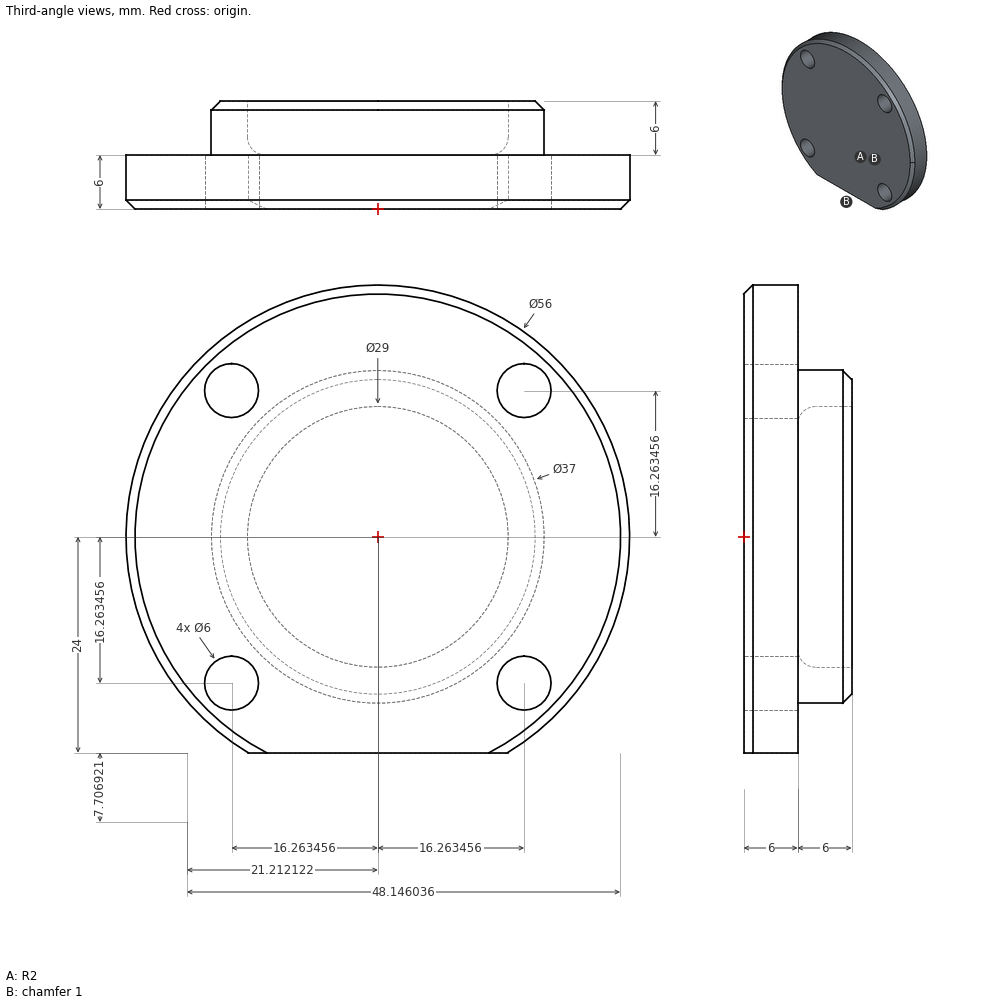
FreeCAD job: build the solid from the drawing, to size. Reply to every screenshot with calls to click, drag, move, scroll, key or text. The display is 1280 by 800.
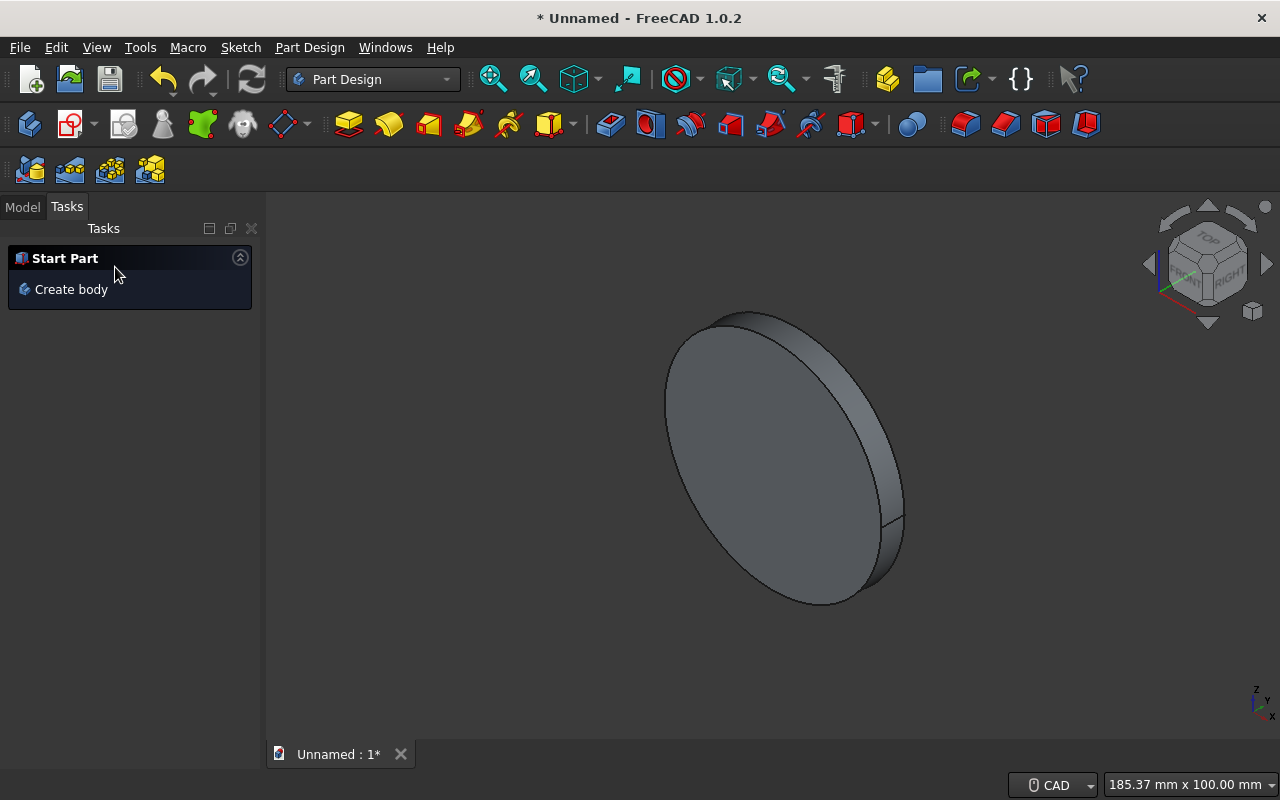
key(2)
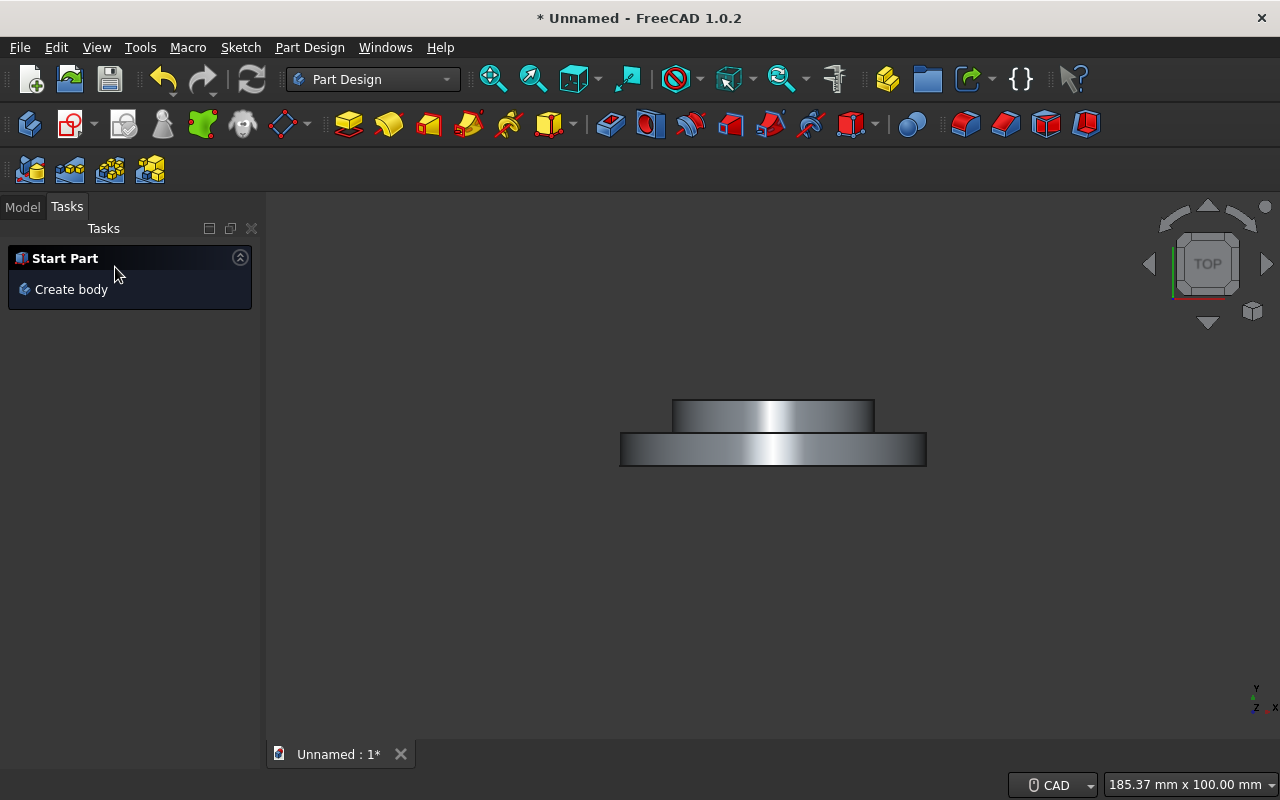
click(494, 80)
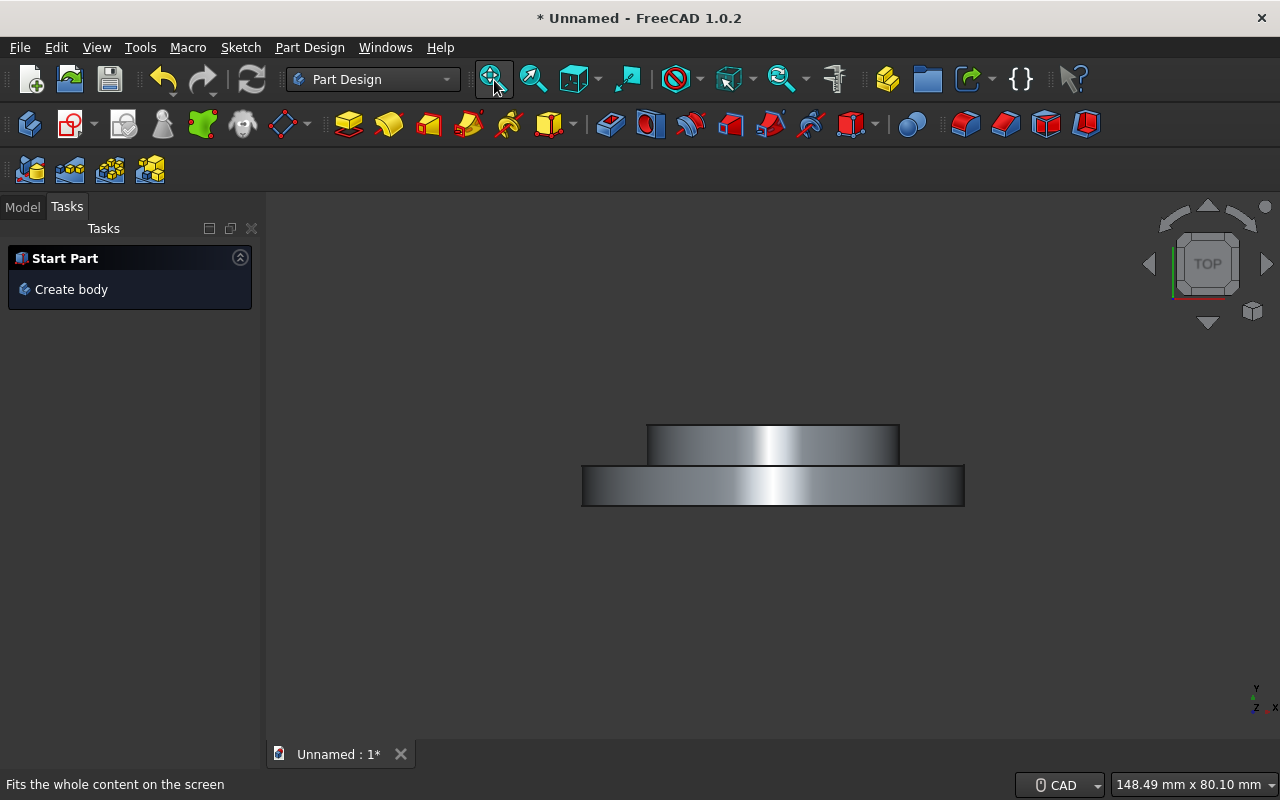
key(1)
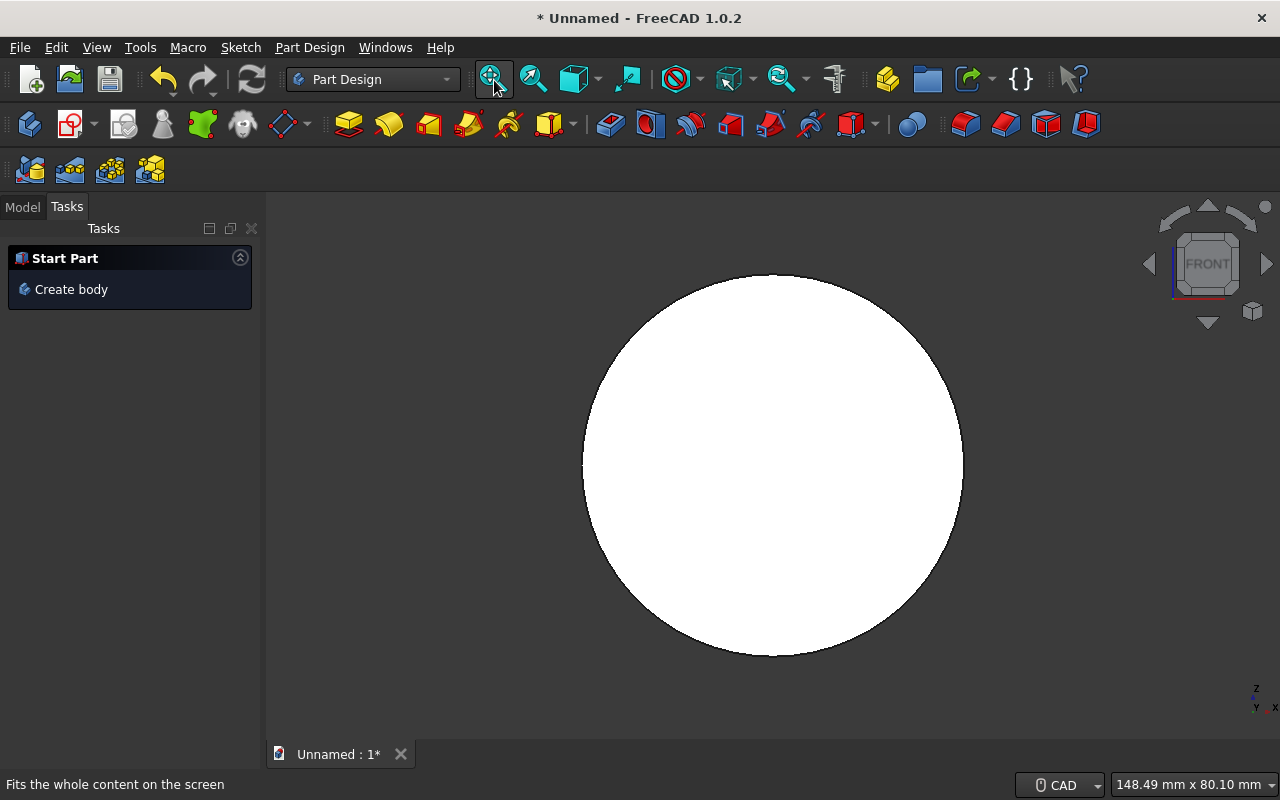
key(3)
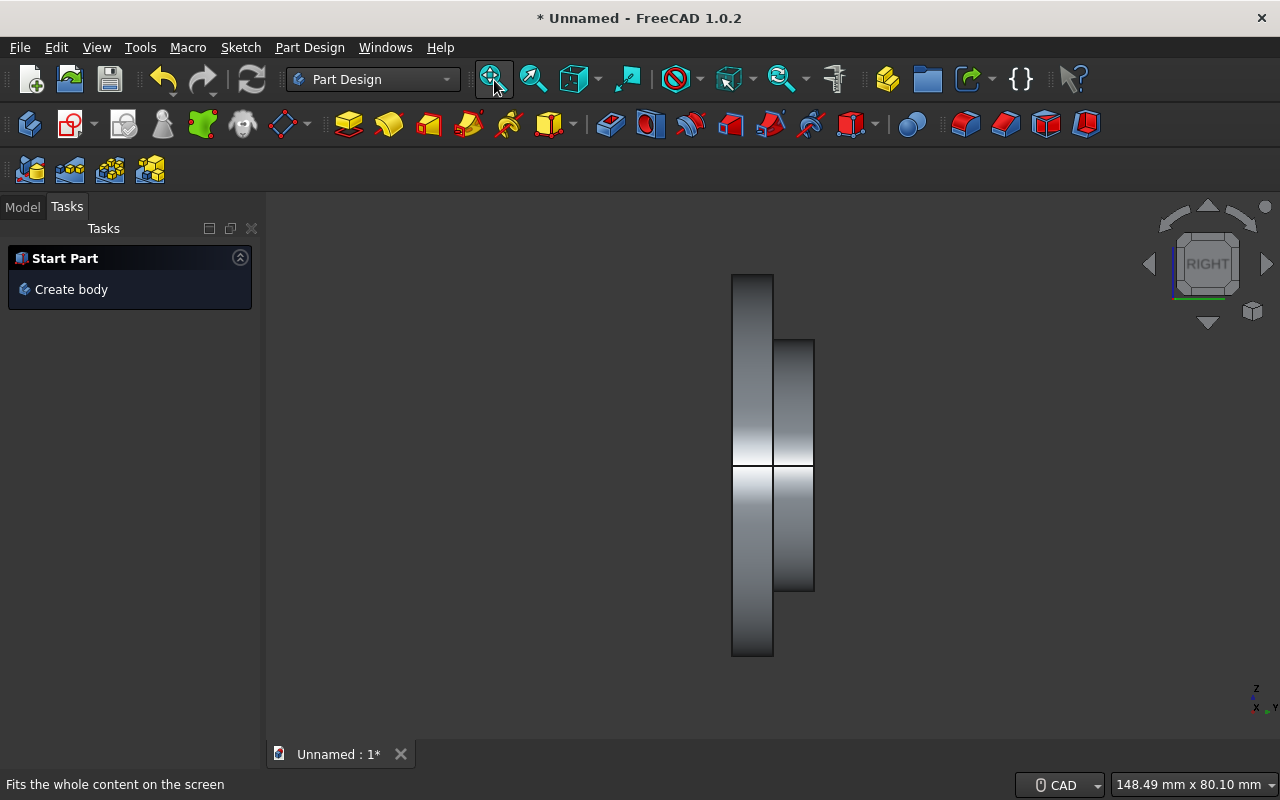
key(5)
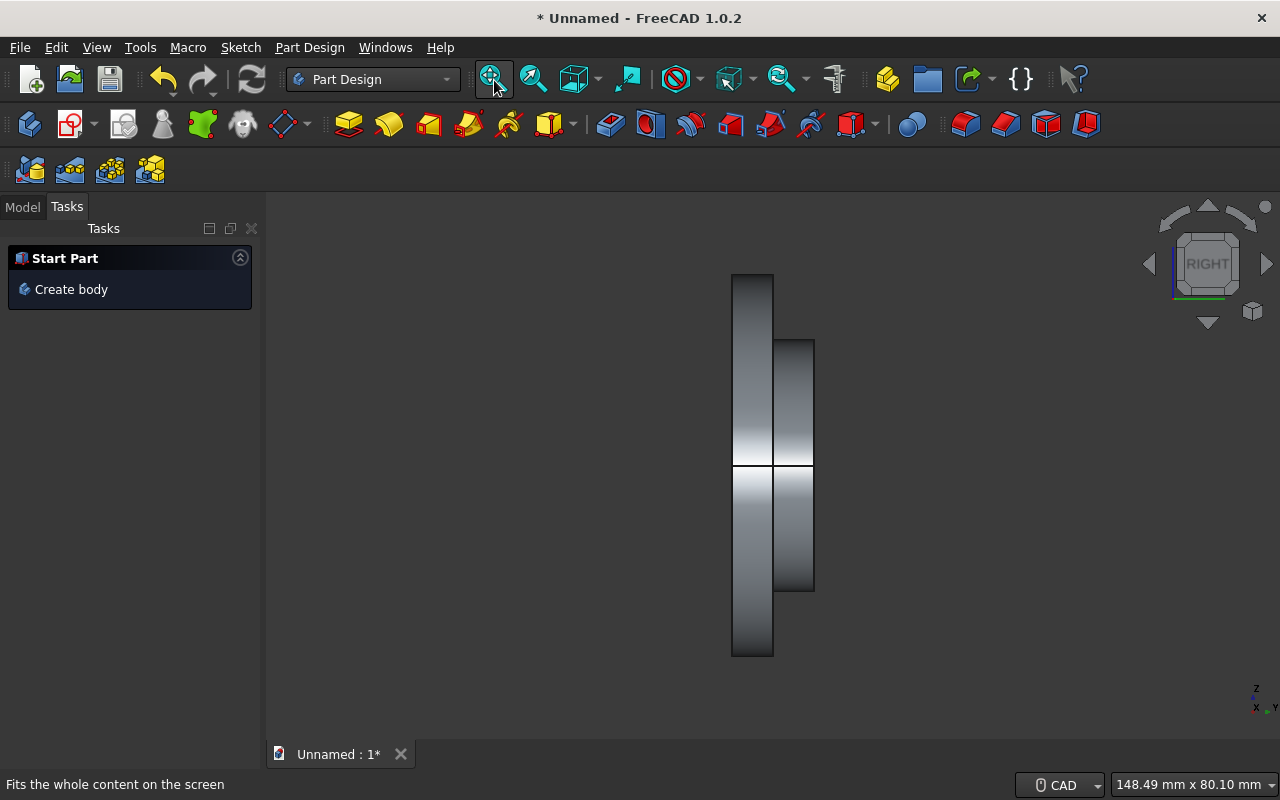
click(494, 80)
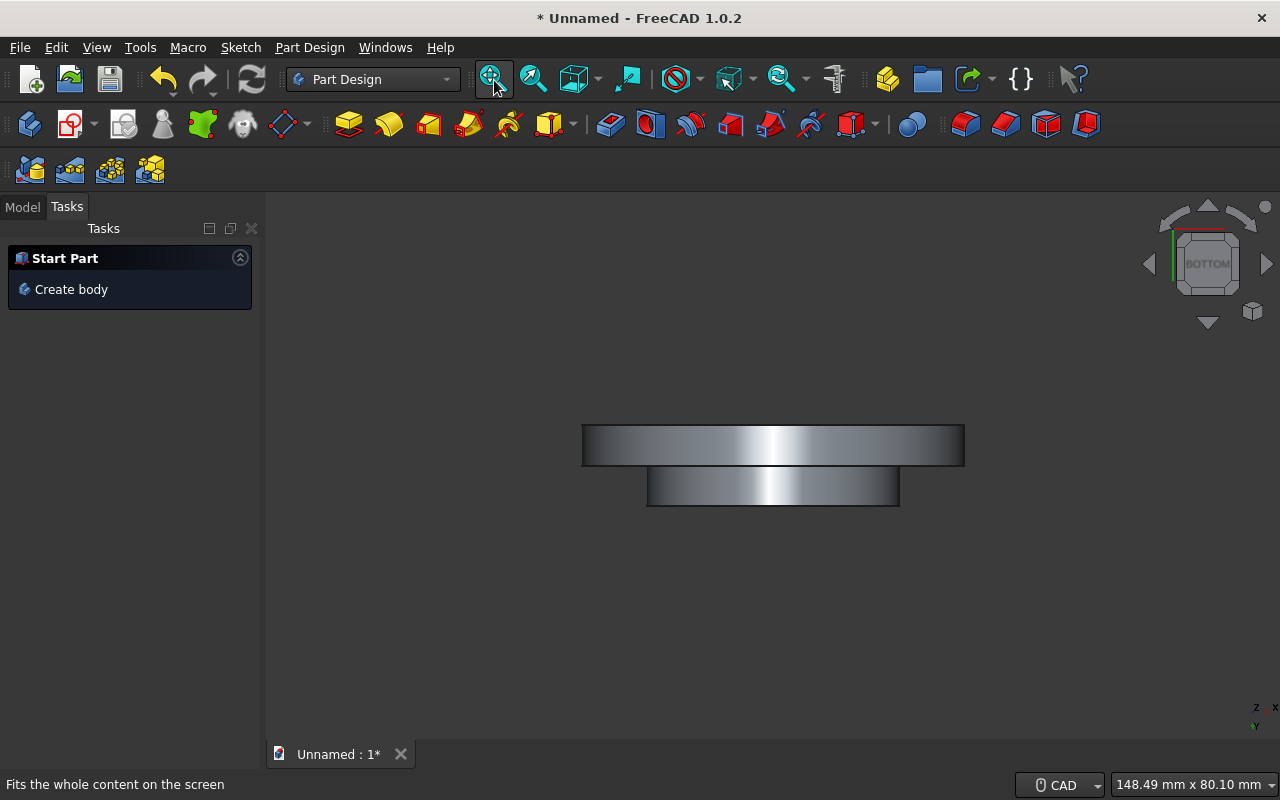
key(4)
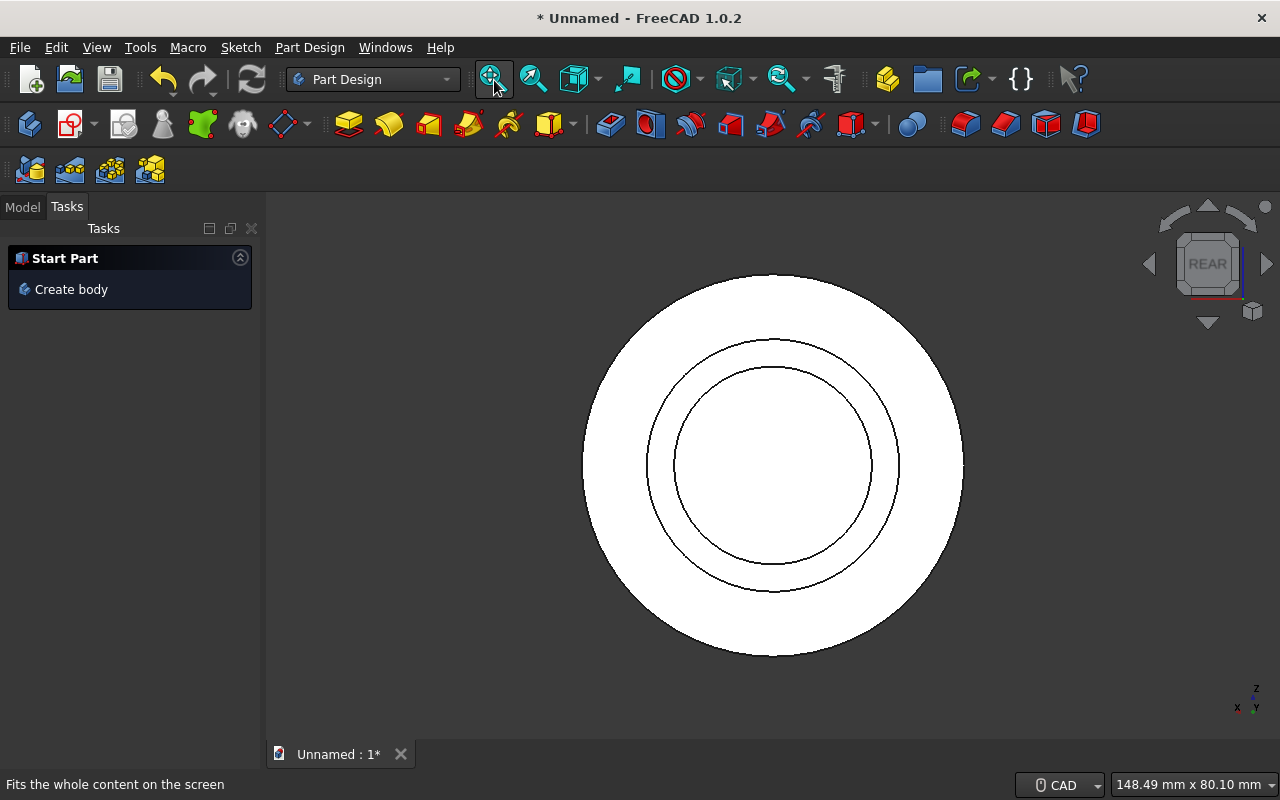
key(6)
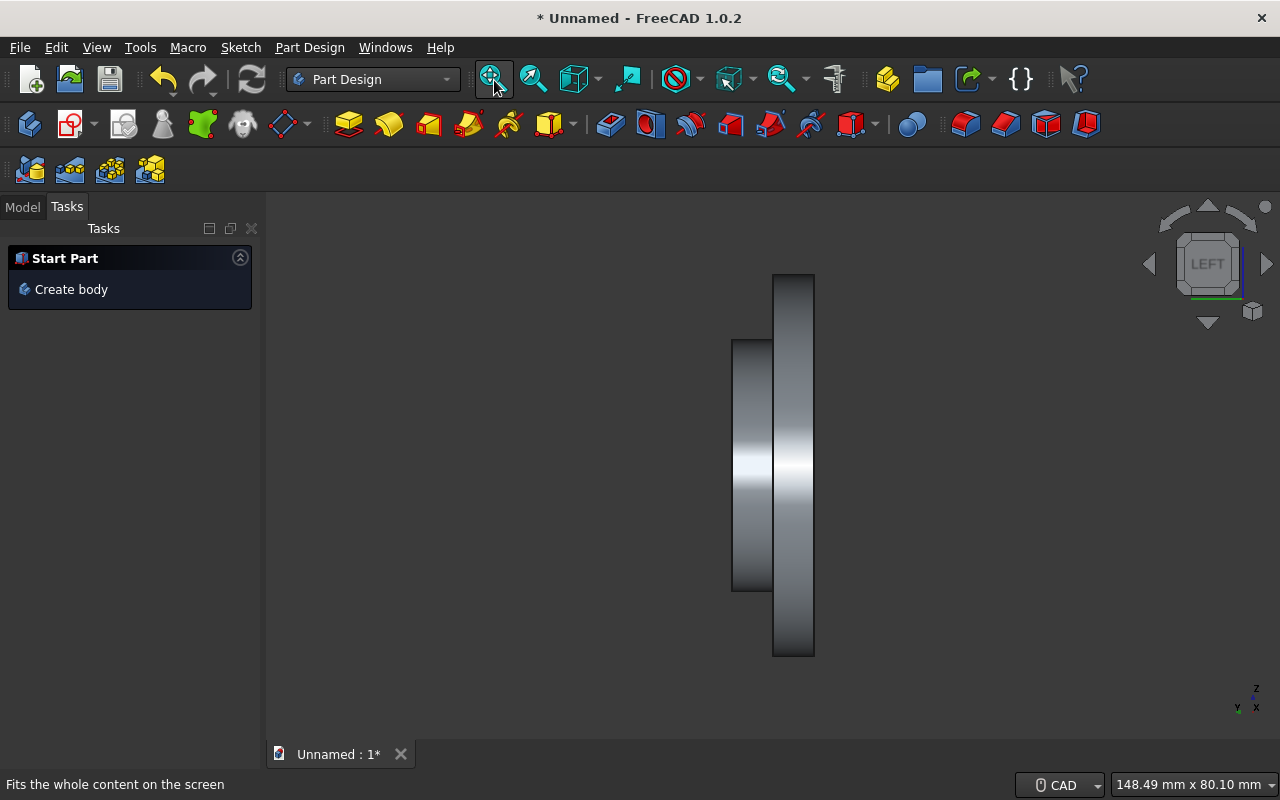
key(v)
key(3)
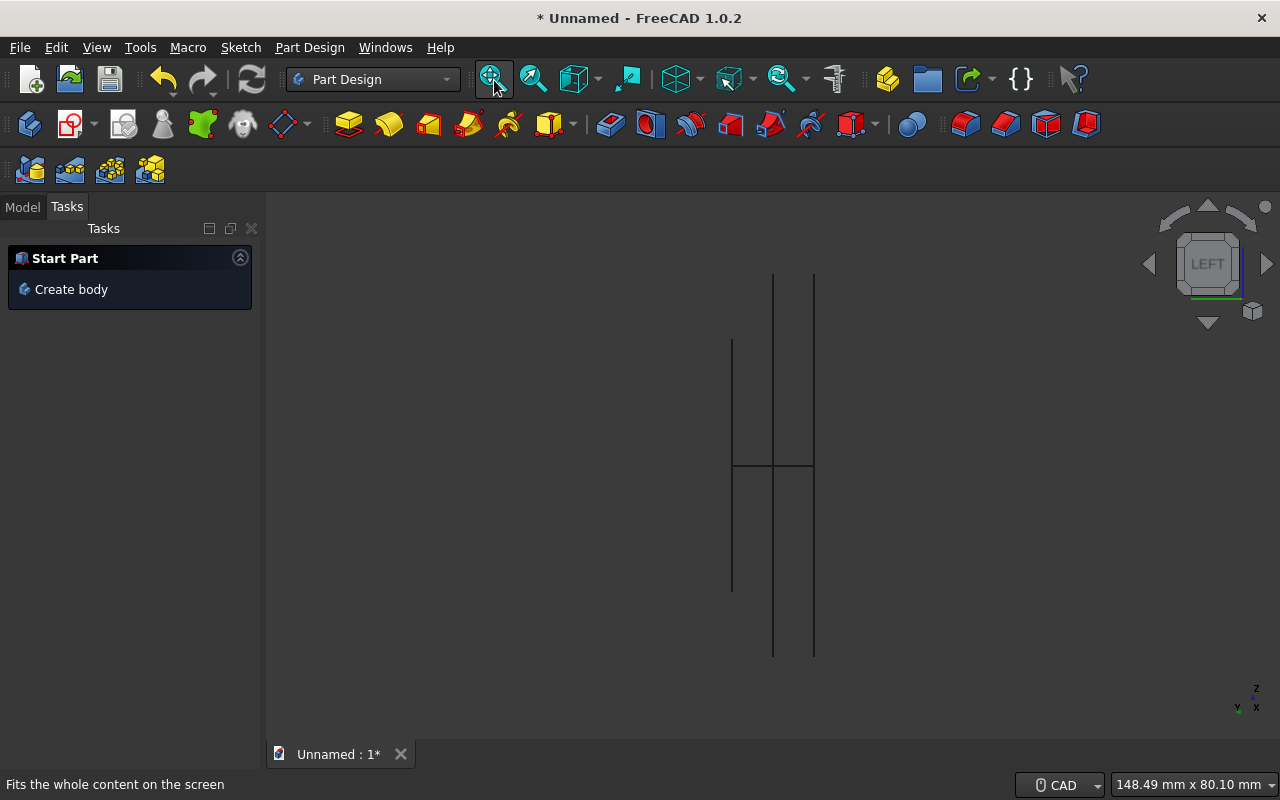
key(0)